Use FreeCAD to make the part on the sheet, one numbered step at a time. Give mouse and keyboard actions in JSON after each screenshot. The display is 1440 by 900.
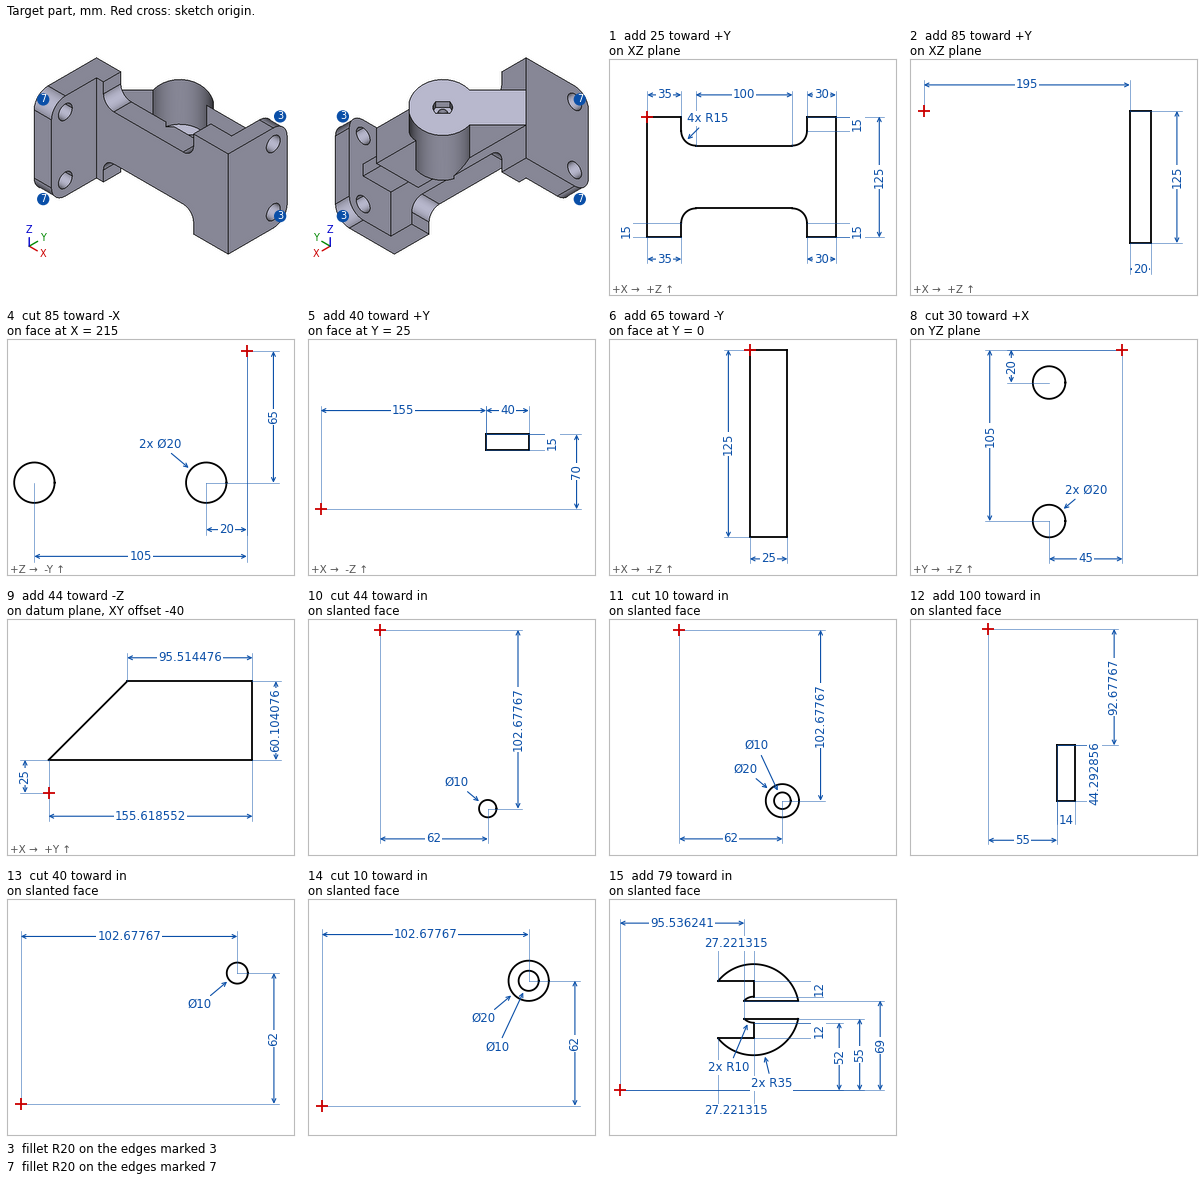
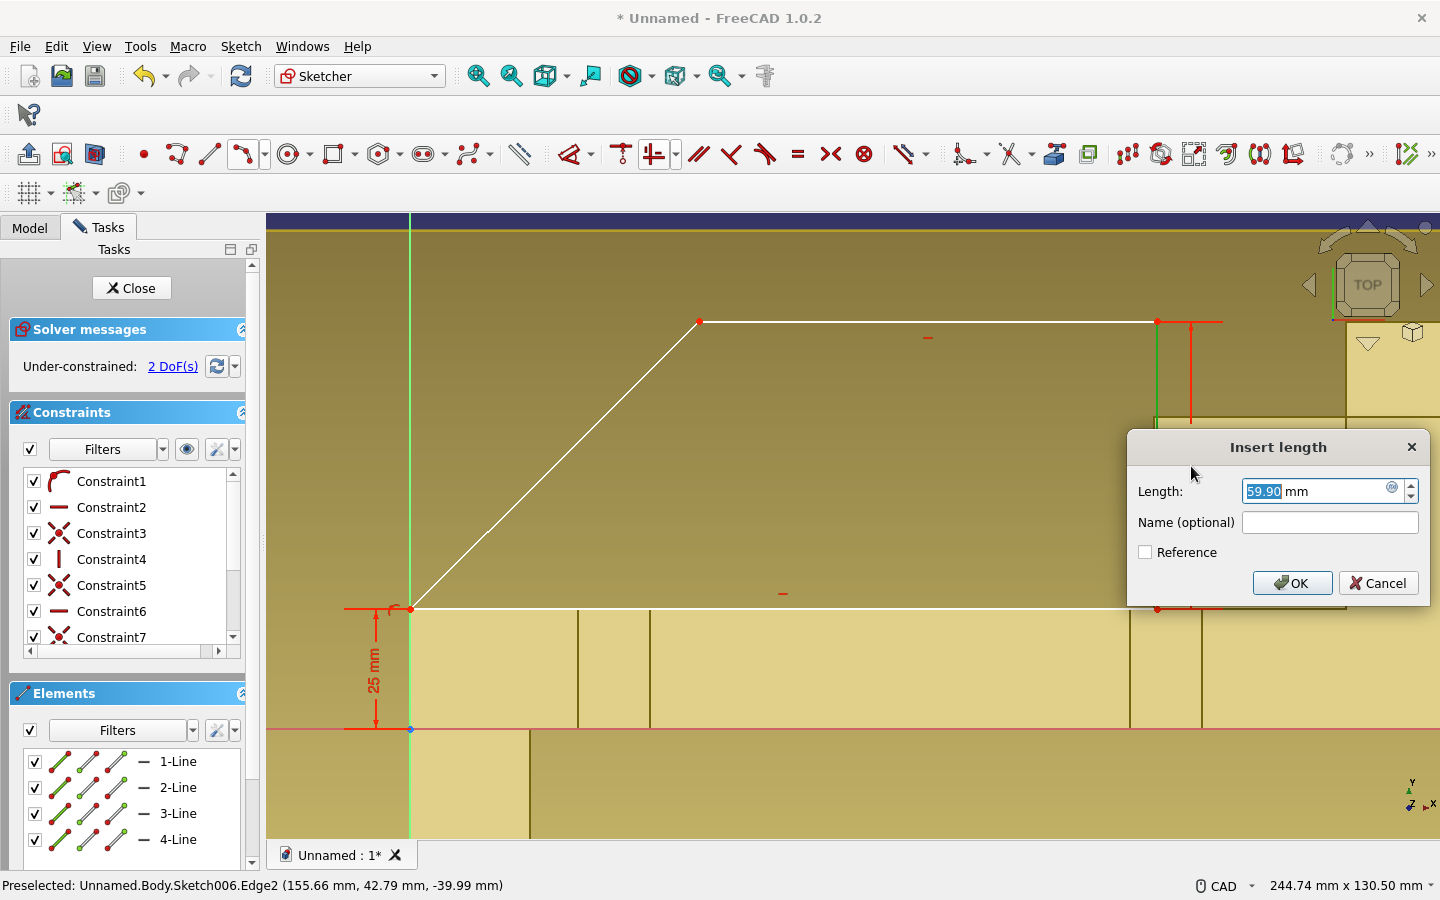
{"action": "type", "text": "60.104076"}
{"action": "key", "text": "Return"}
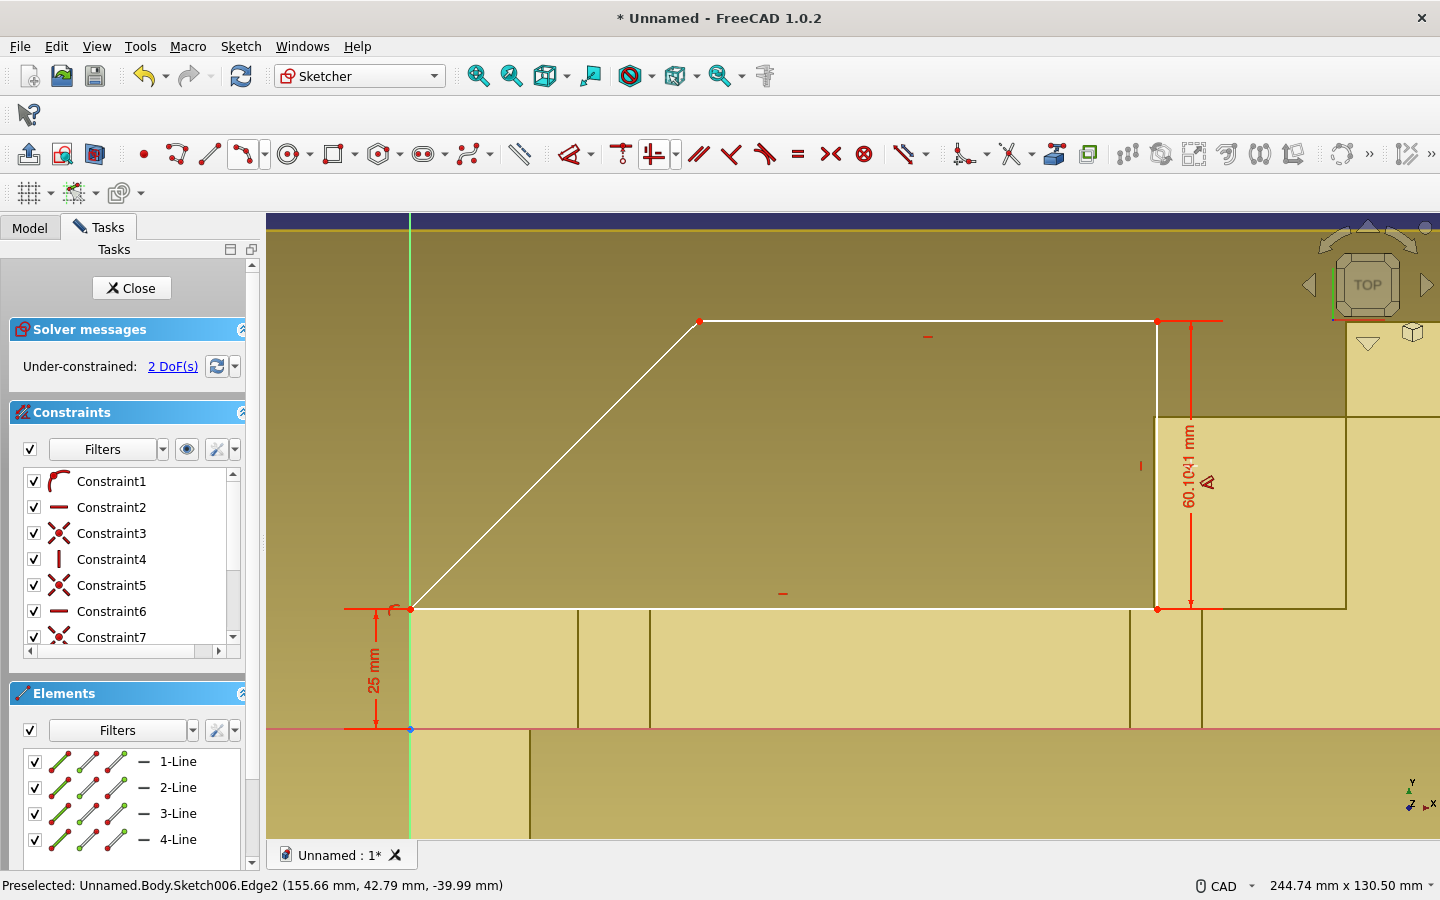
{"action": "left_click", "coordinate": [1020, 321]}
{"action": "left_click", "coordinate": [928, 287]}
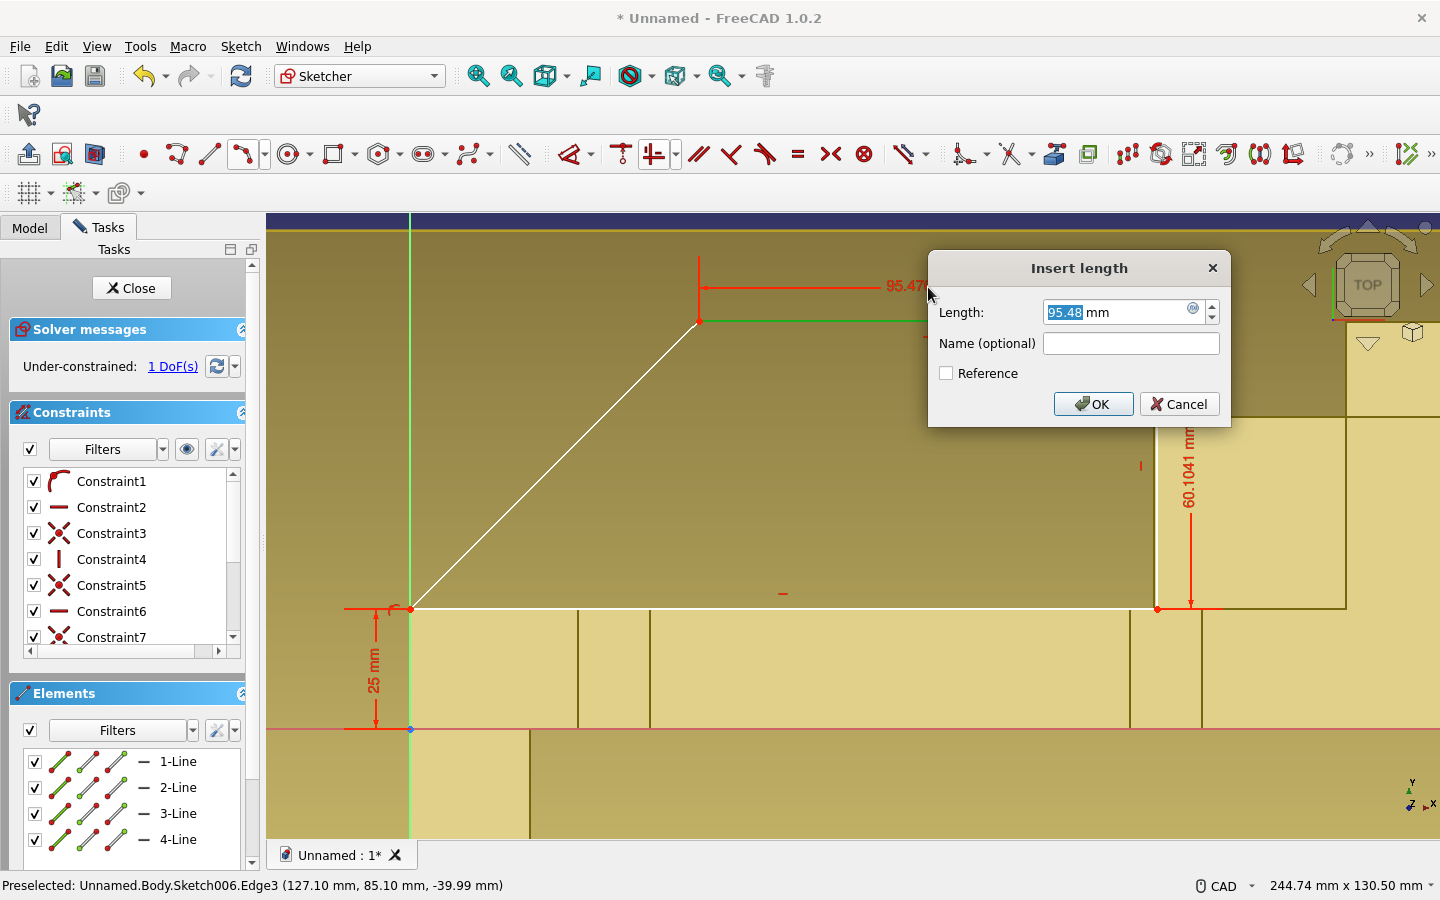
{"action": "type", "text": "95.514476"}
{"action": "key", "text": "Return"}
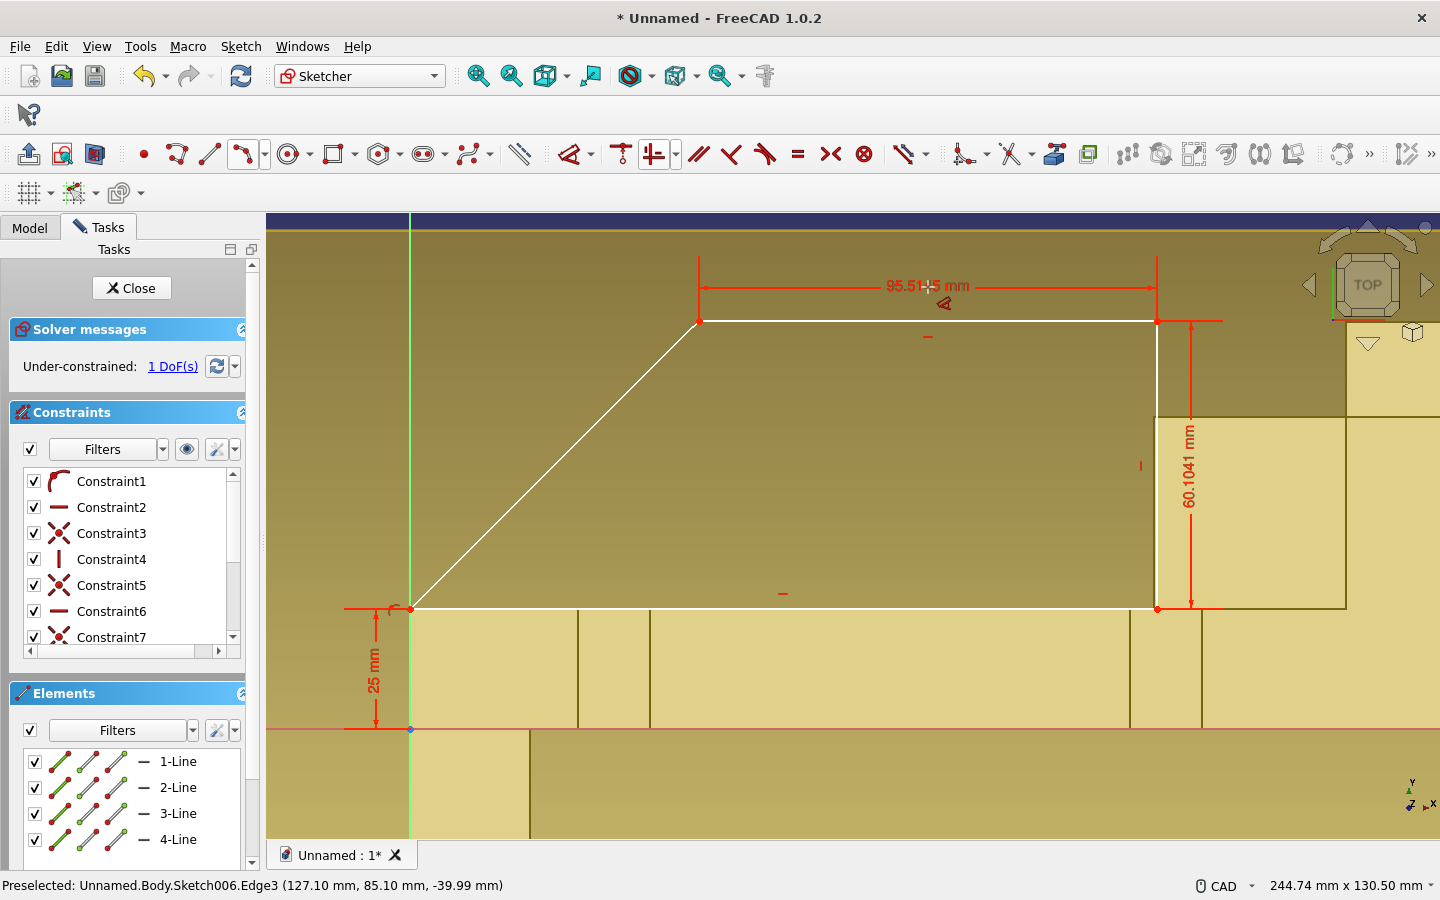
{"action": "left_click", "coordinate": [634, 609]}
{"action": "left_click", "coordinate": [784, 643]}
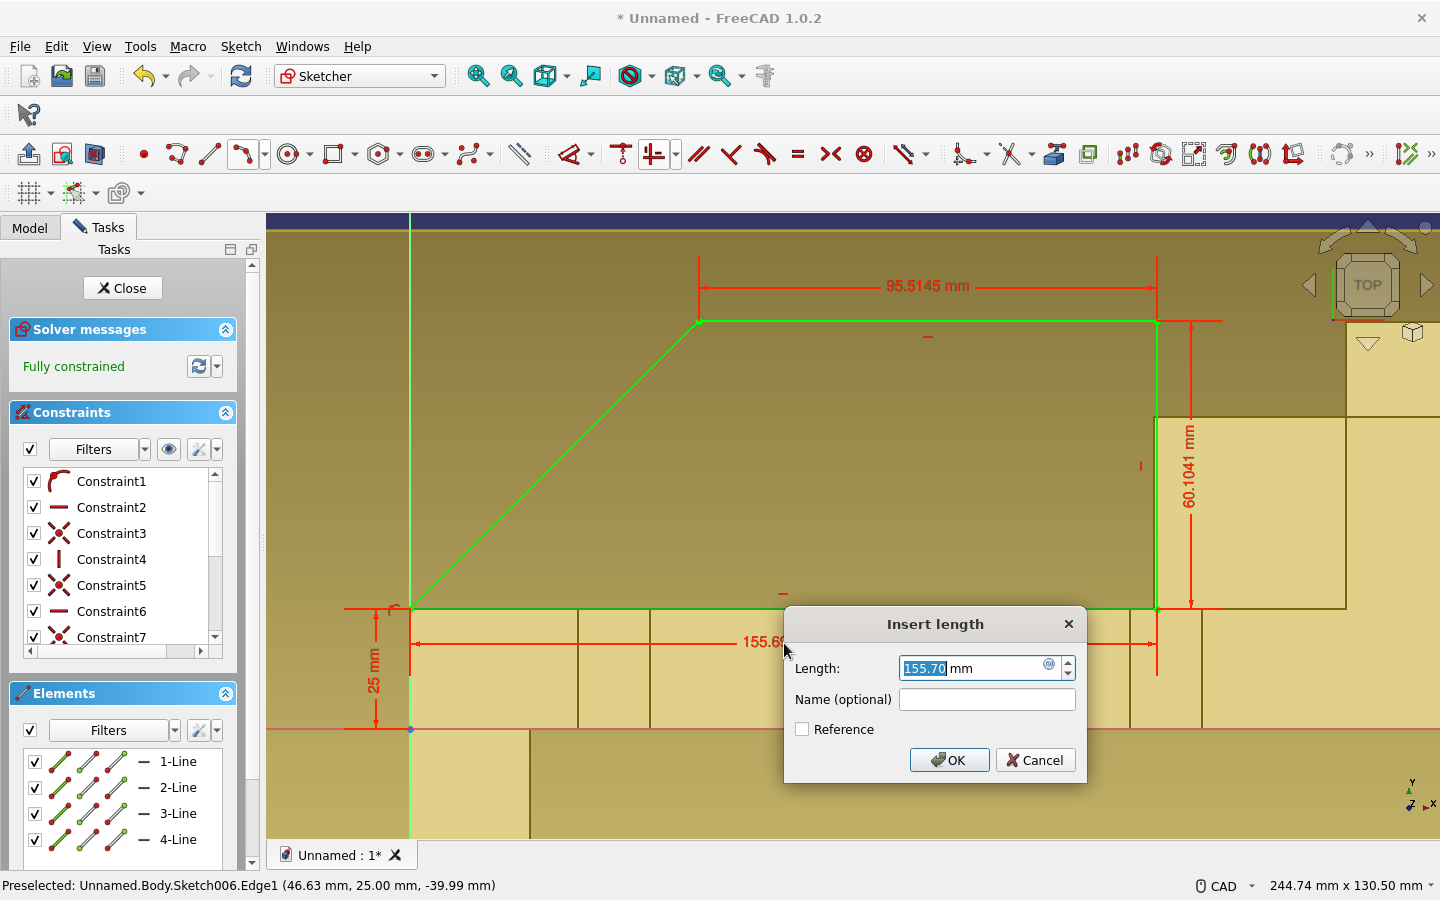
{"action": "type", "text": "155.618552"}
{"action": "key", "text": "Return"}
{"action": "key", "text": "Escape"}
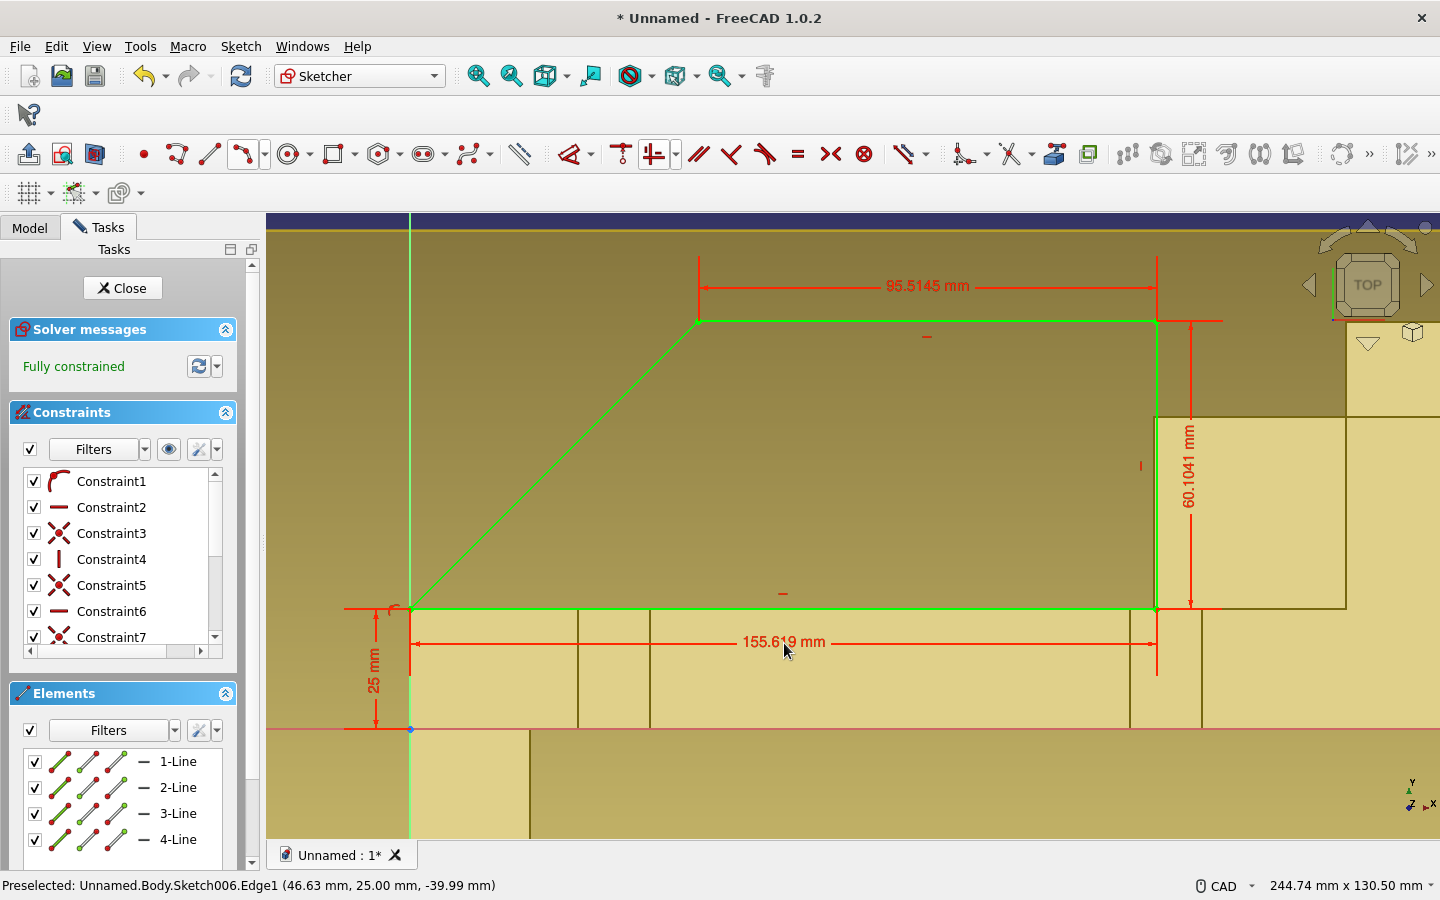
{"action": "left_click", "coordinate": [123, 288]}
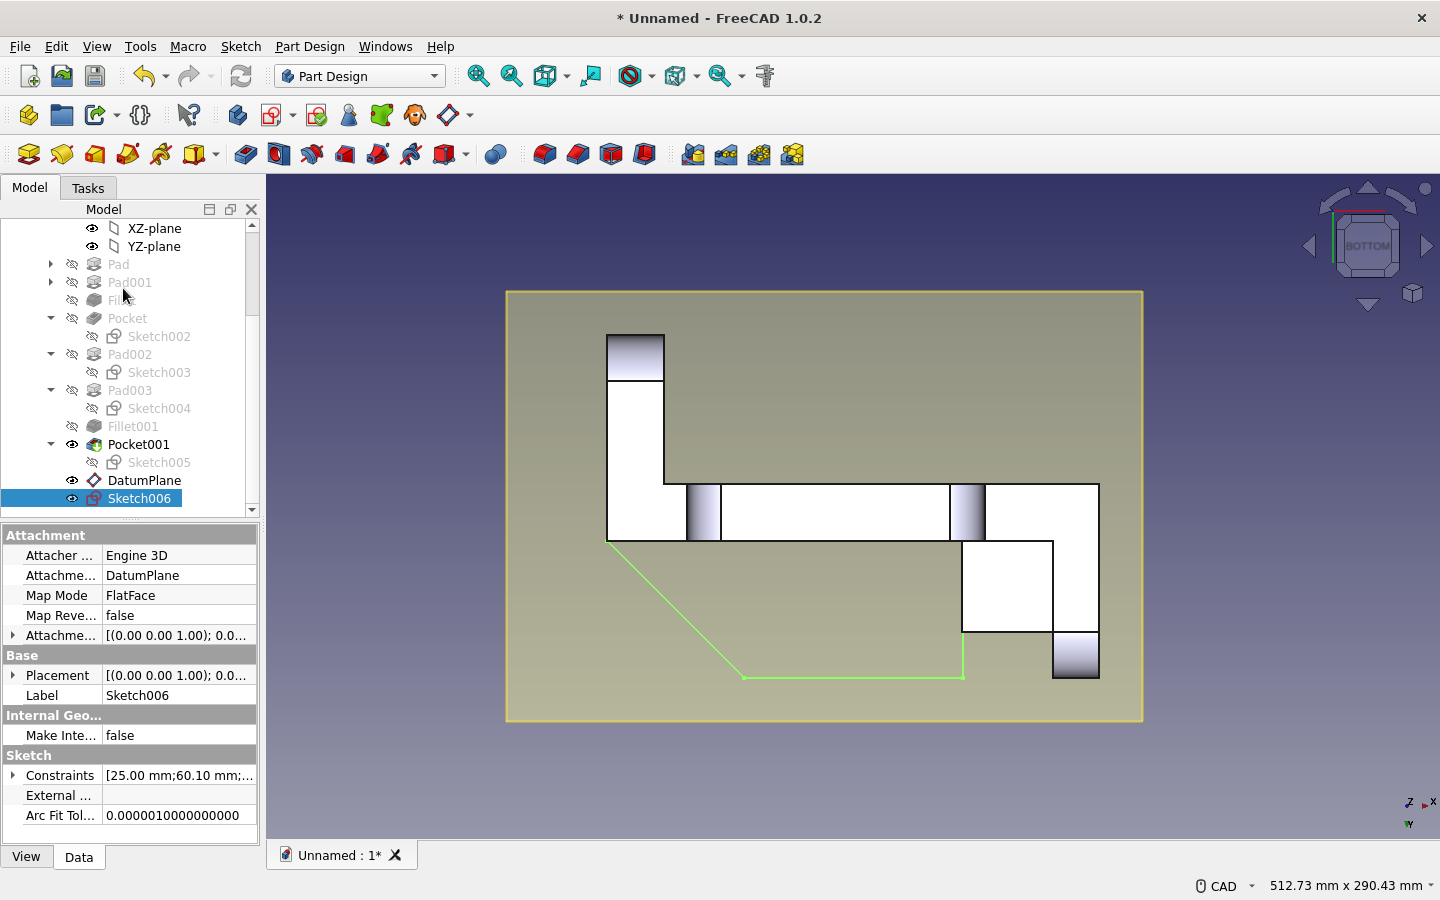
{"action": "left_click", "coordinate": [29, 154]}